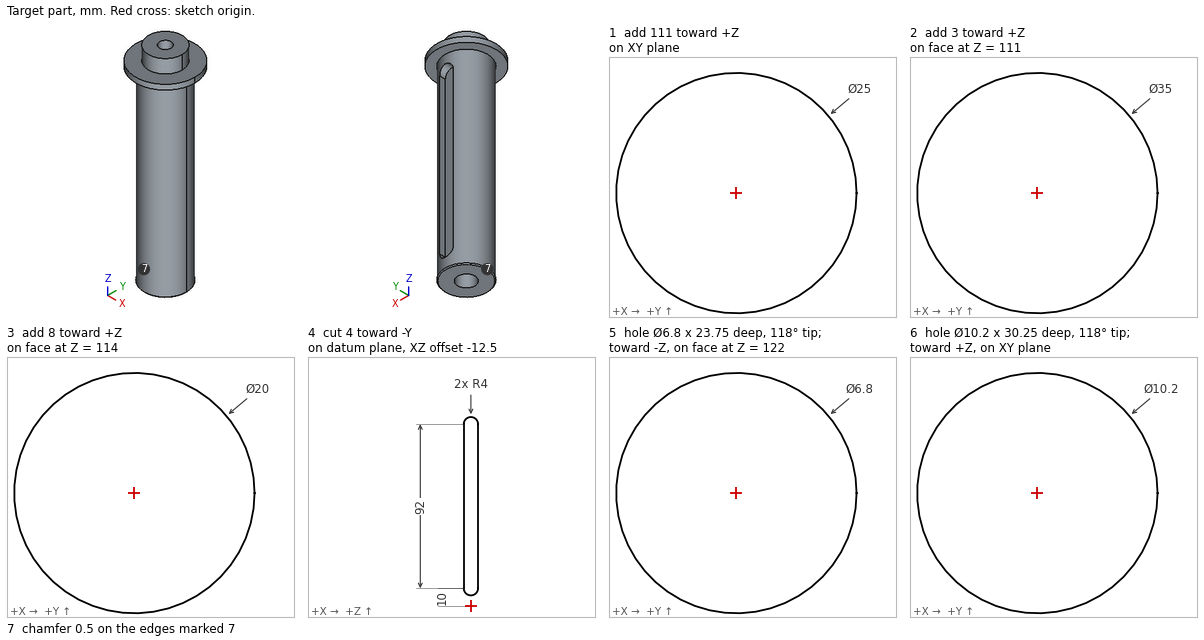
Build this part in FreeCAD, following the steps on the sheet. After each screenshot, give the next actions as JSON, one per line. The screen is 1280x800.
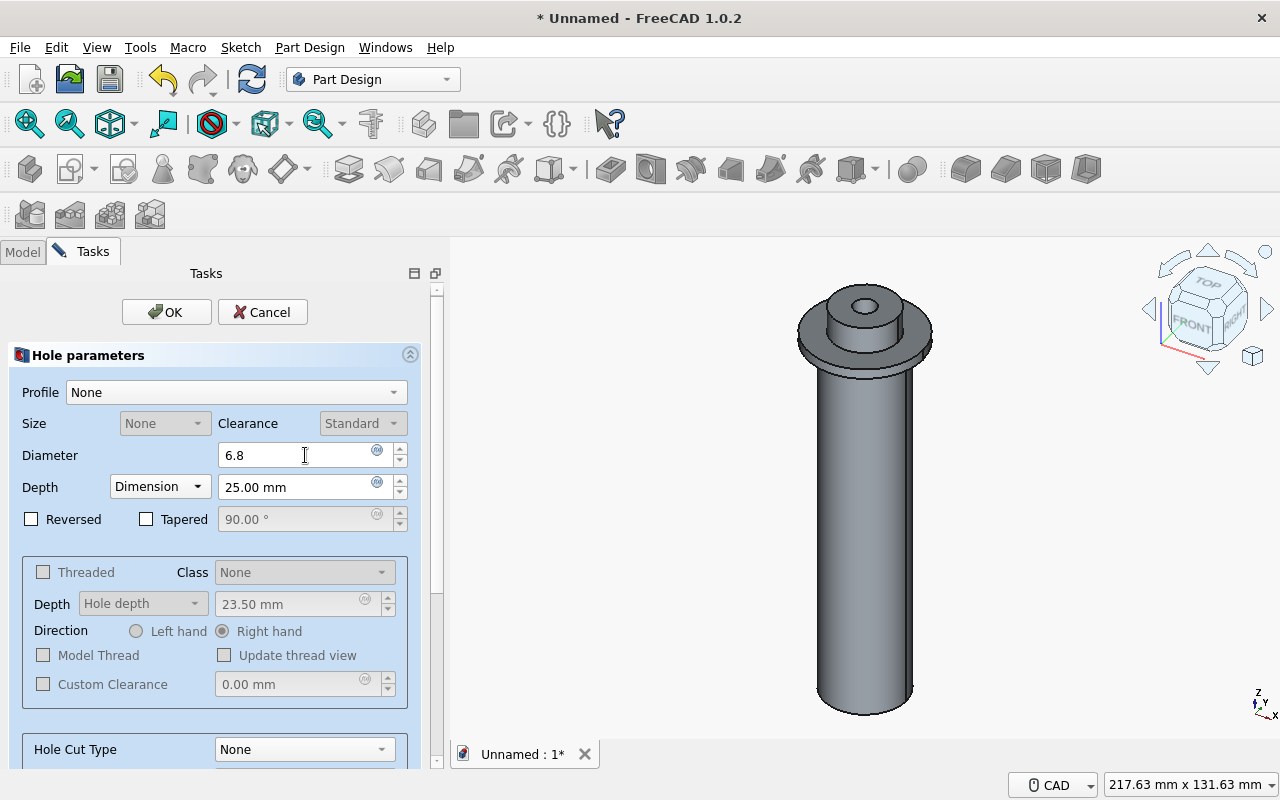
{"action": "triple_click", "coordinate": [305, 487]}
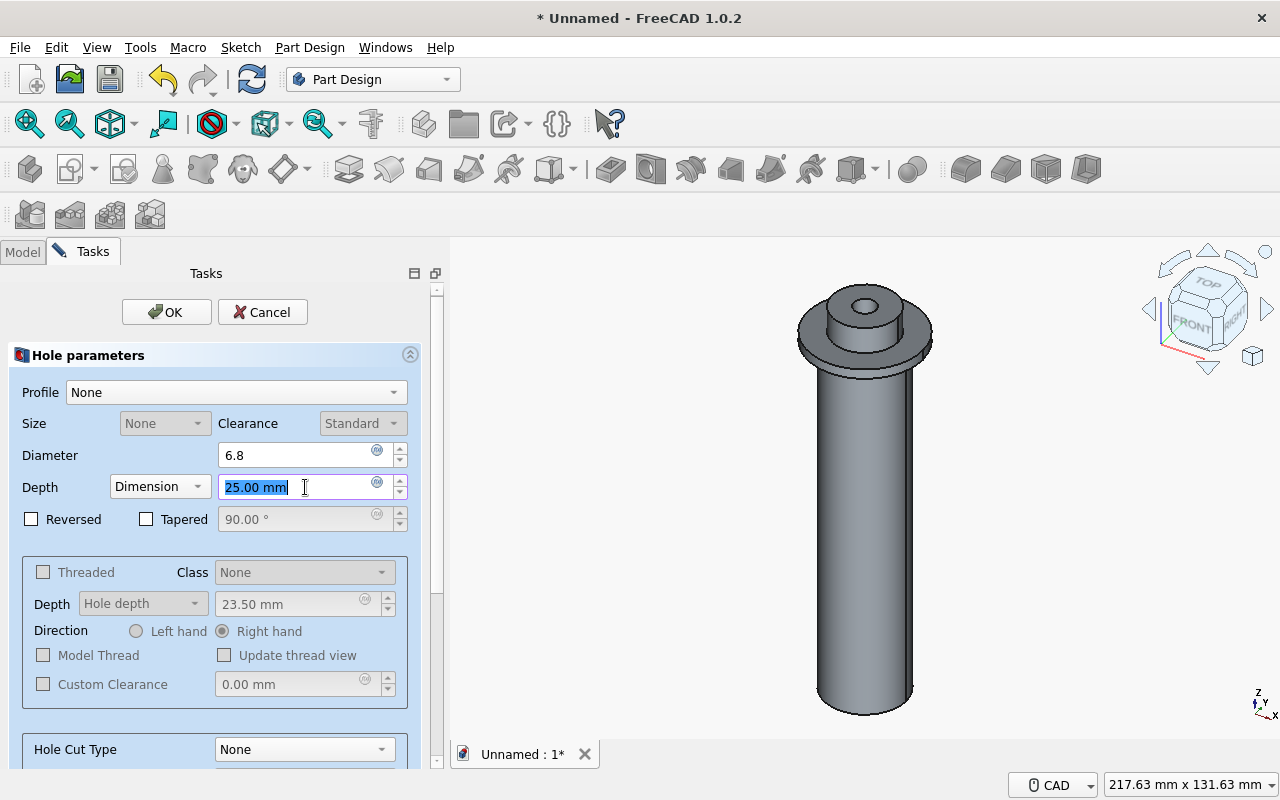
{"action": "type", "text": "23.75"}
{"action": "key", "text": "Tab"}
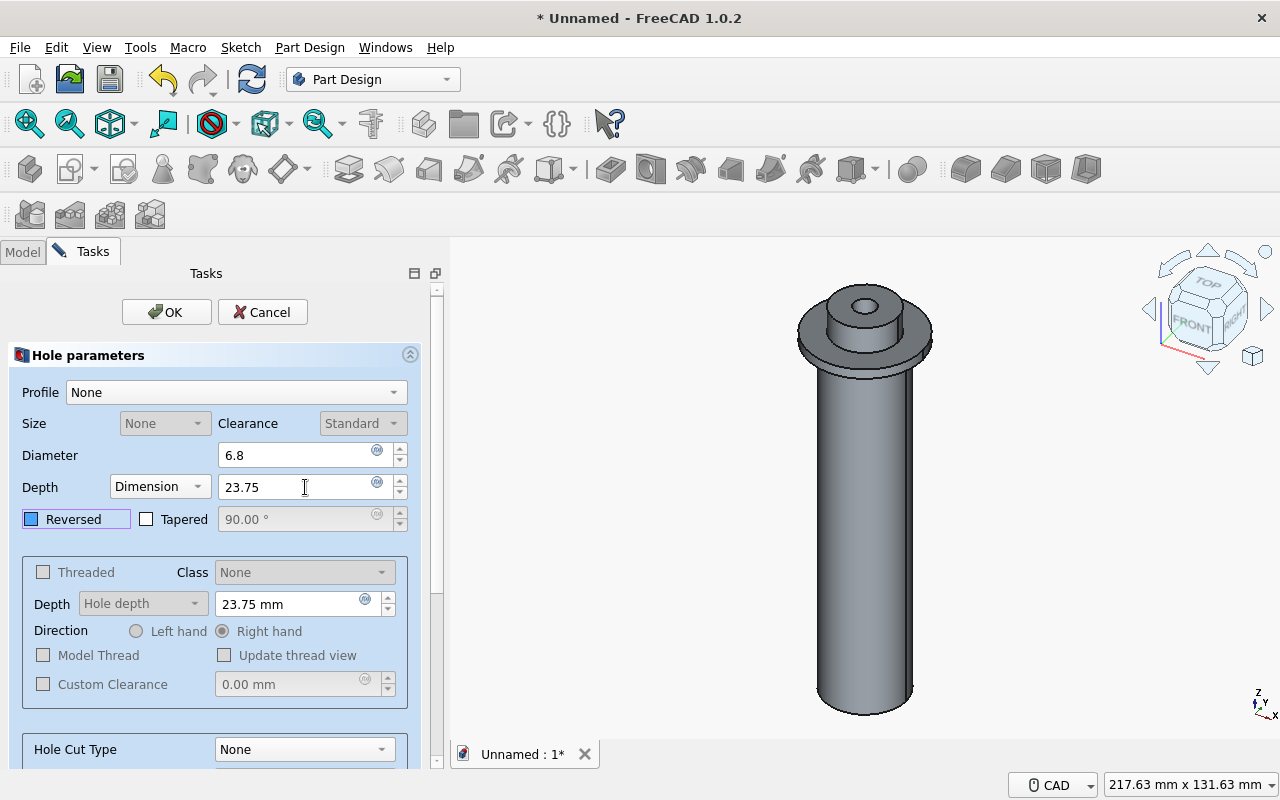
{"action": "left_click", "coordinate": [167, 312]}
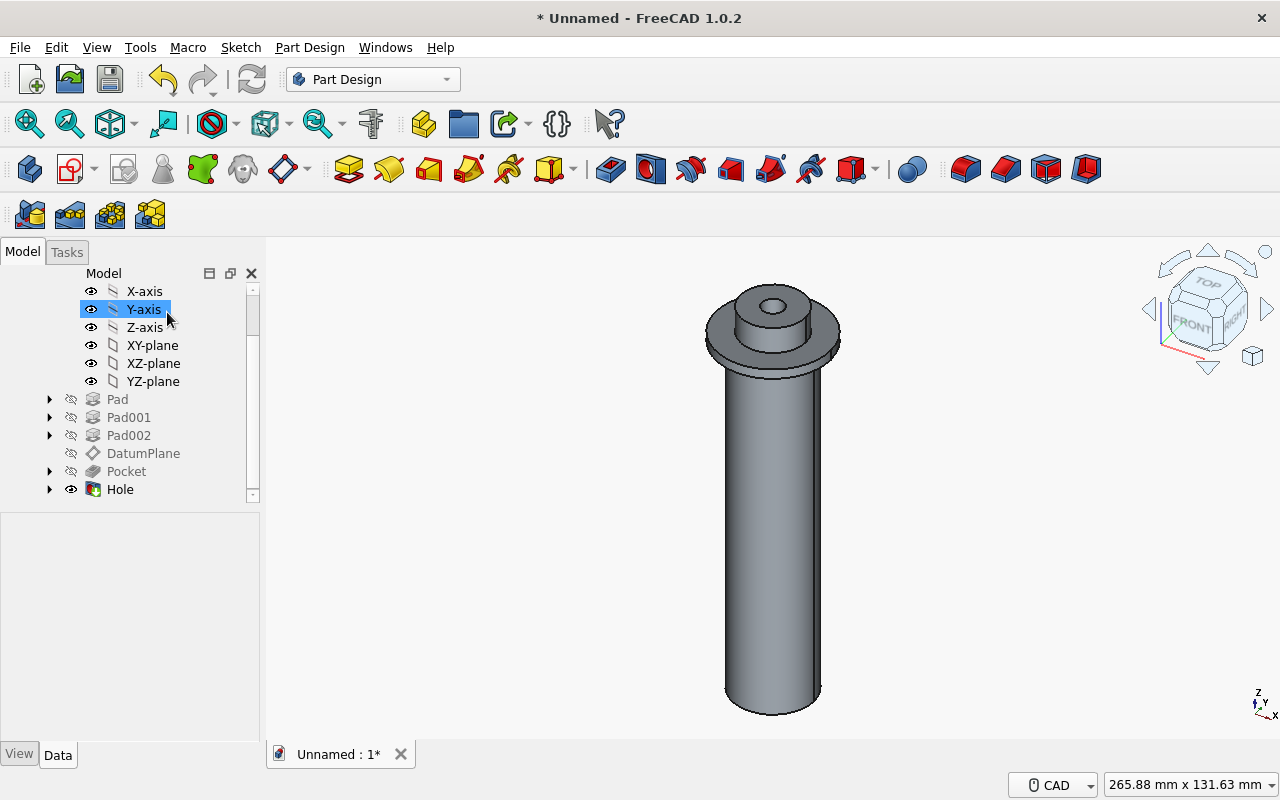
{"action": "left_click", "coordinate": [70, 170]}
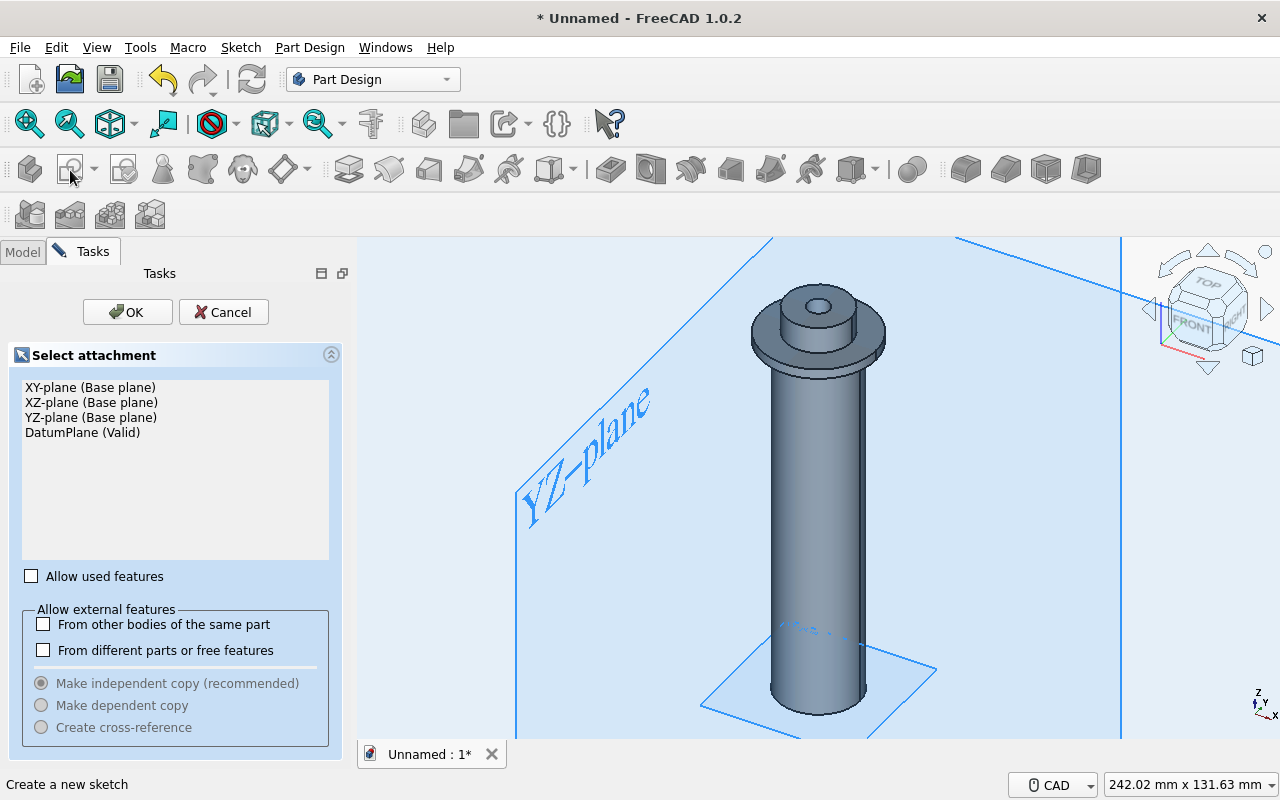
{"action": "left_click", "coordinate": [82, 388]}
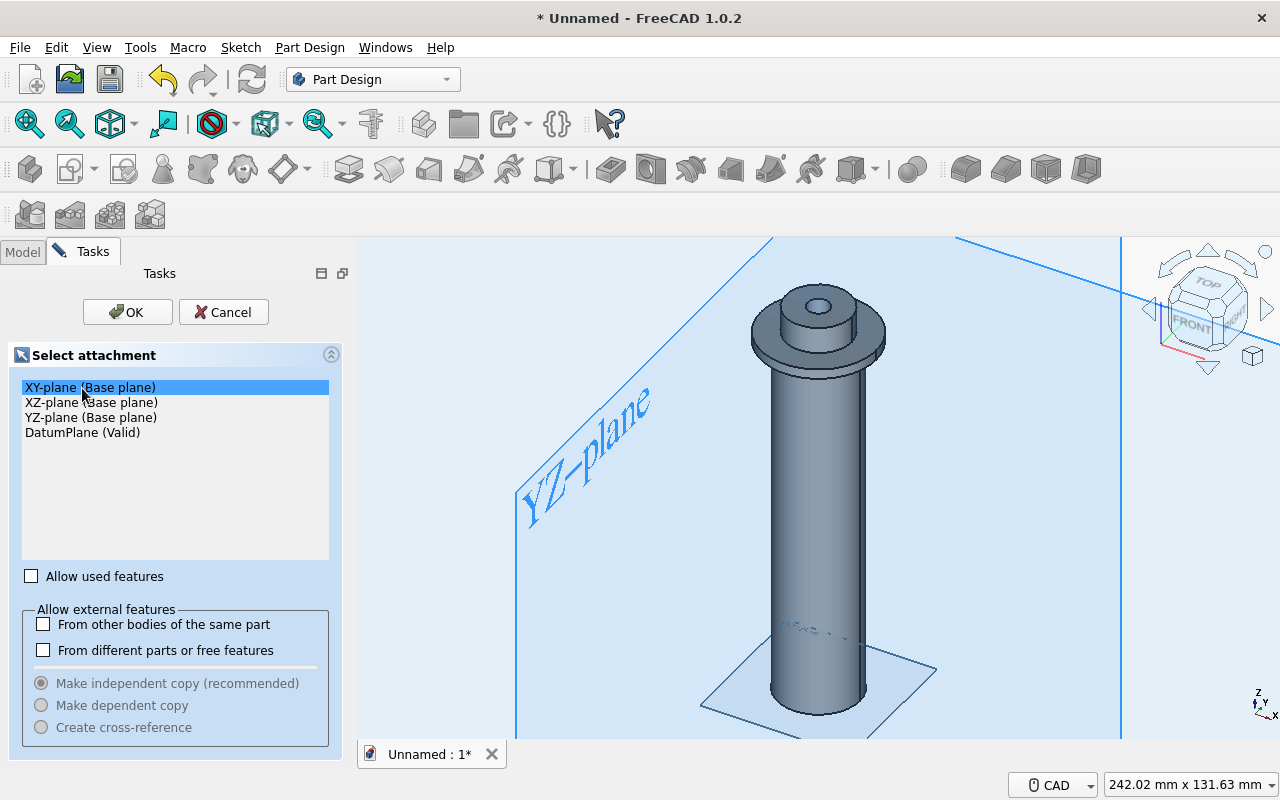
{"action": "left_click", "coordinate": [128, 312]}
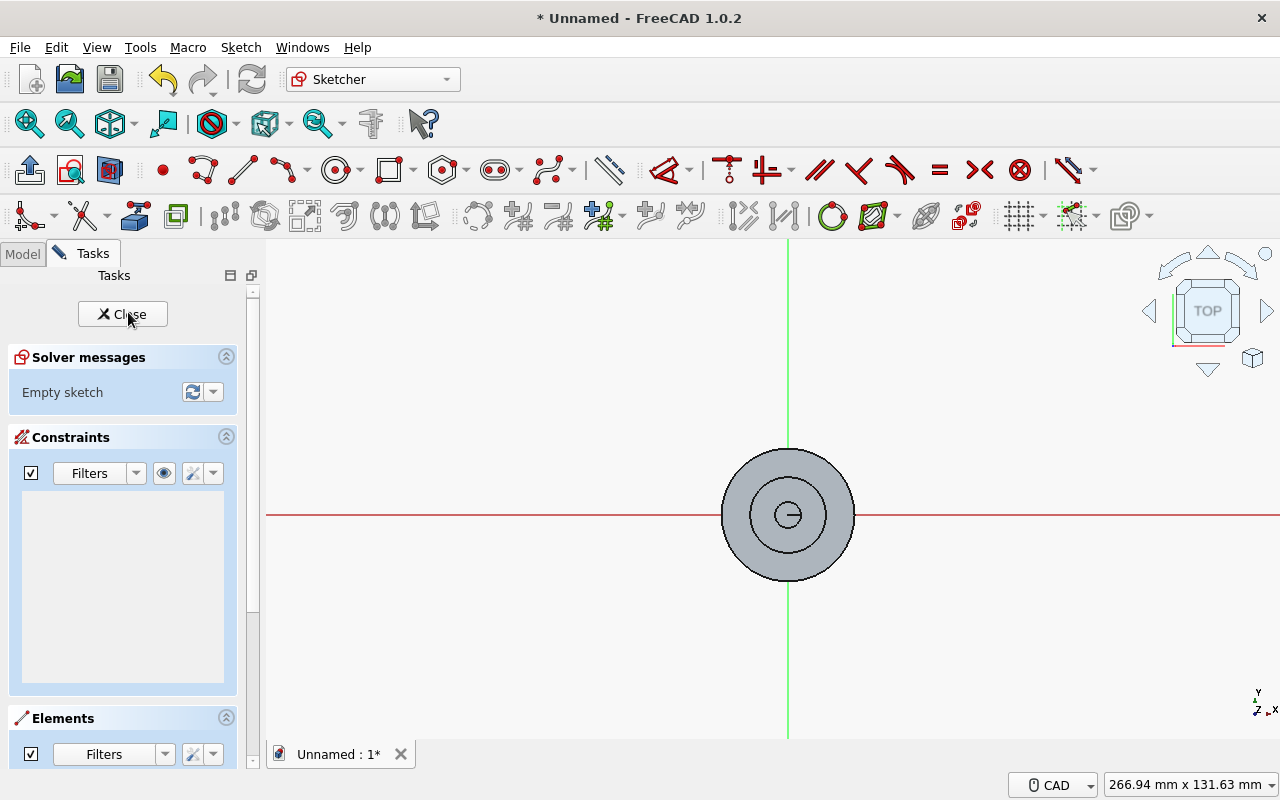
{"action": "left_click", "coordinate": [110, 170]}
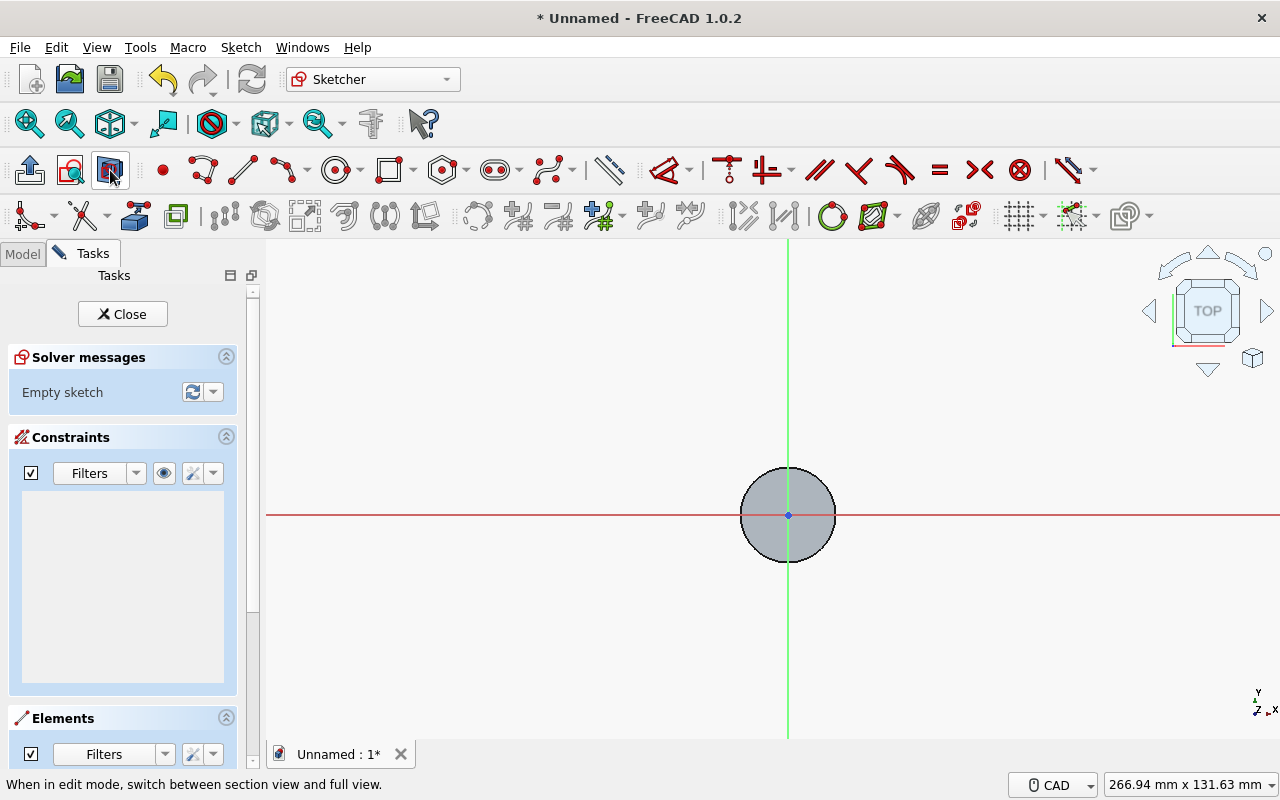
{"action": "scroll", "coordinate": [801, 519], "scroll_direction": "up", "scroll_amount": 10}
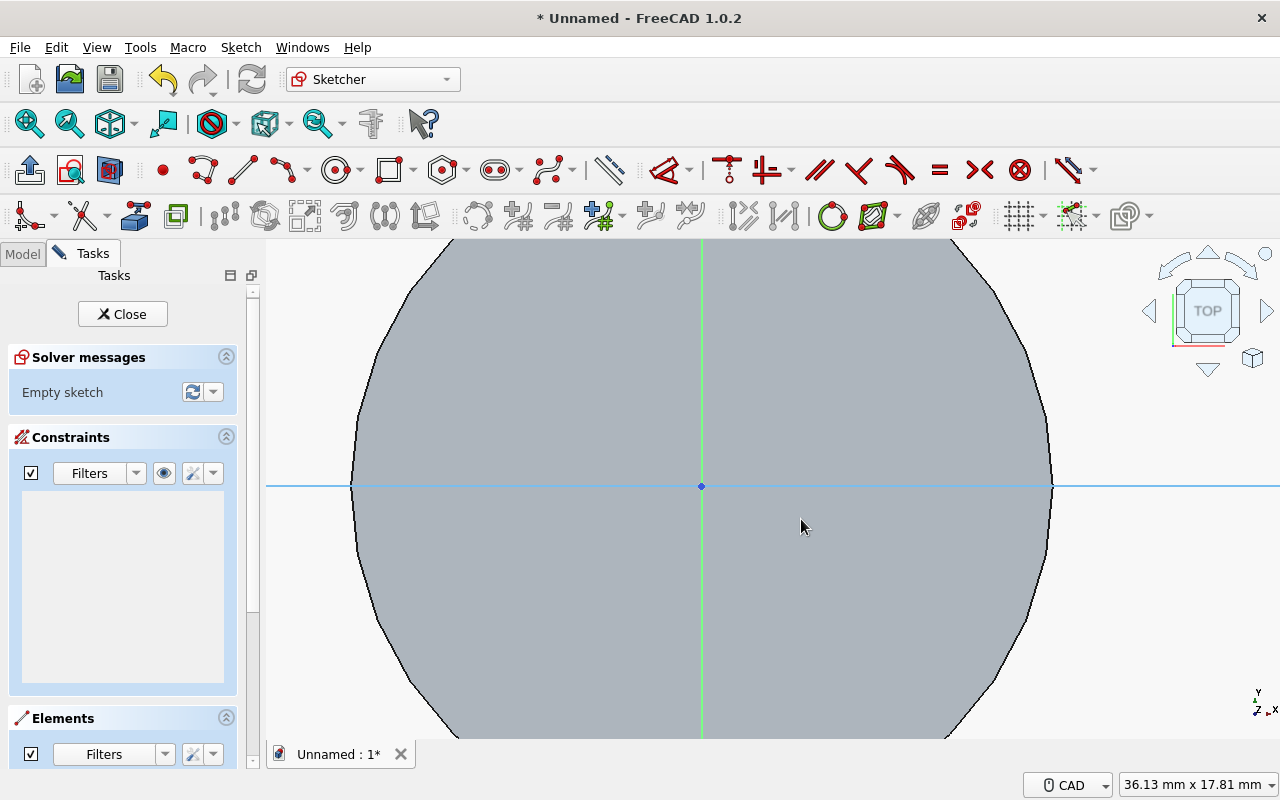
{"action": "left_click", "coordinate": [336, 170]}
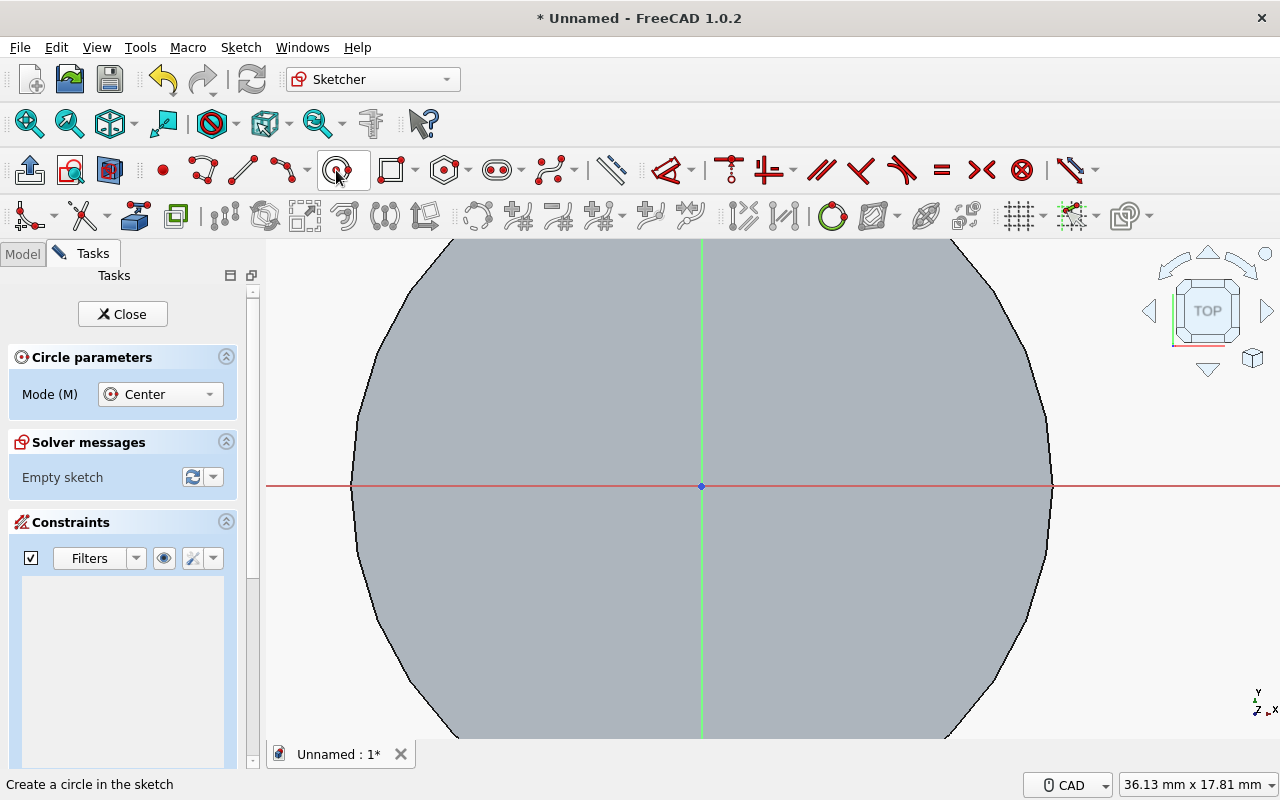
{"action": "left_click", "coordinate": [702, 486]}
{"action": "mouse_move", "coordinate": [803, 385]}